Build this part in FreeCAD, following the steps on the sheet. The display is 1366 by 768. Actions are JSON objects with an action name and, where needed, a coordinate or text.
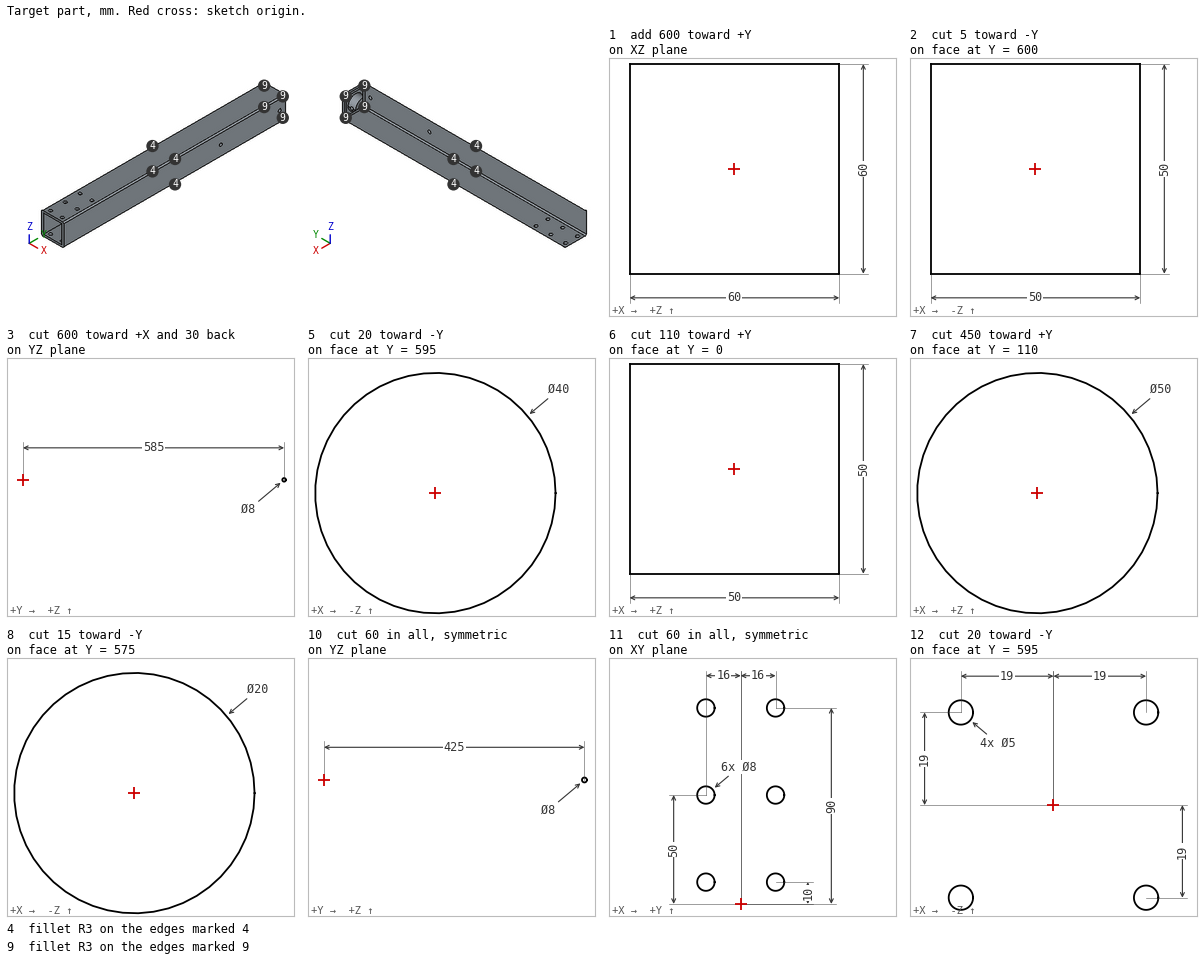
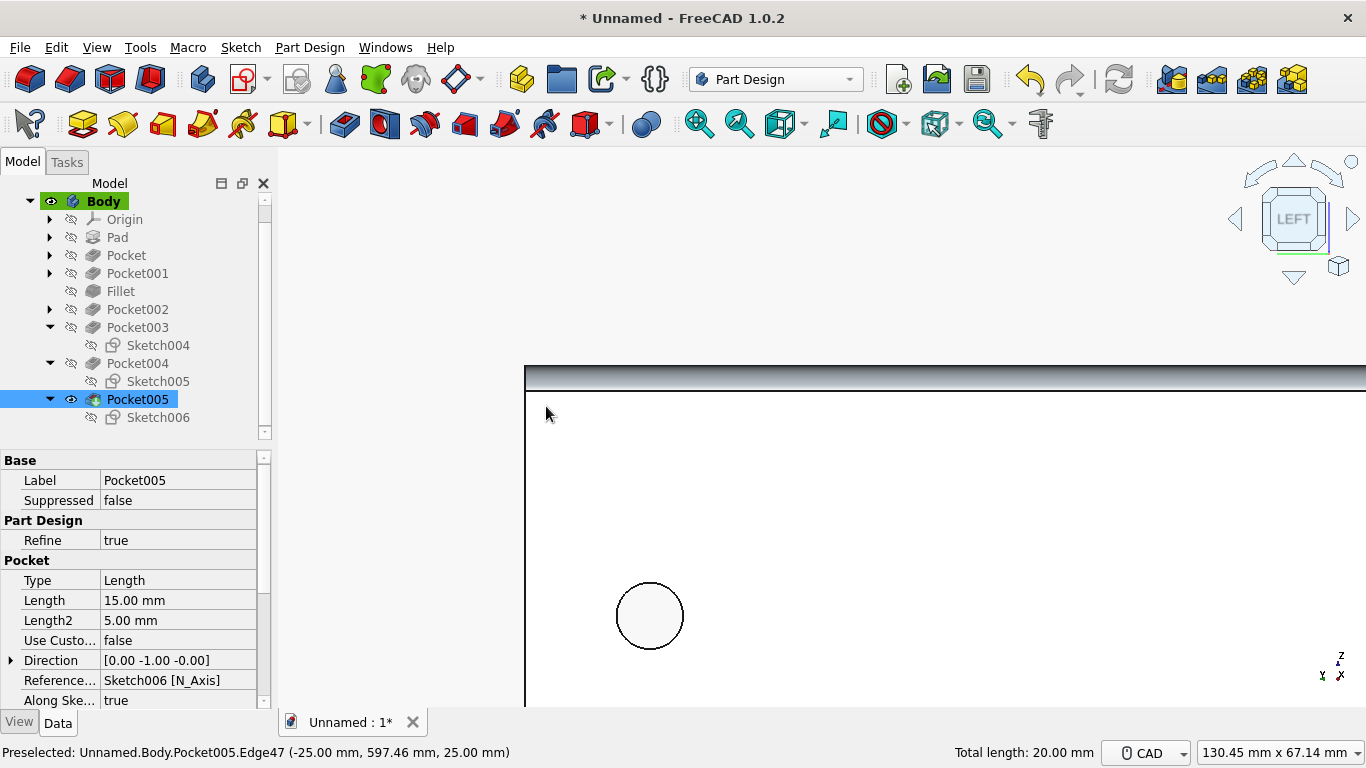
{"action": "left_click", "coordinate": [30, 80]}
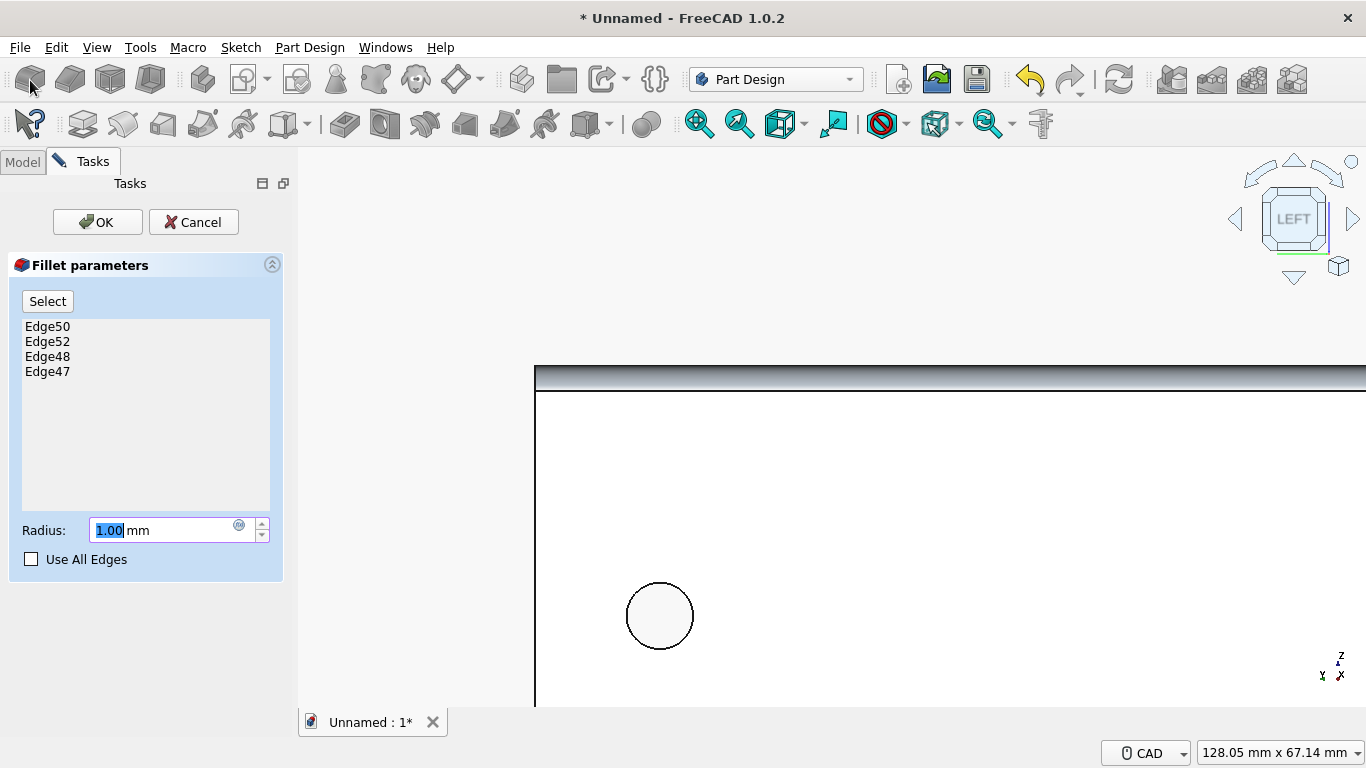
{"action": "type", "text": "3"}
{"action": "key", "text": "Tab"}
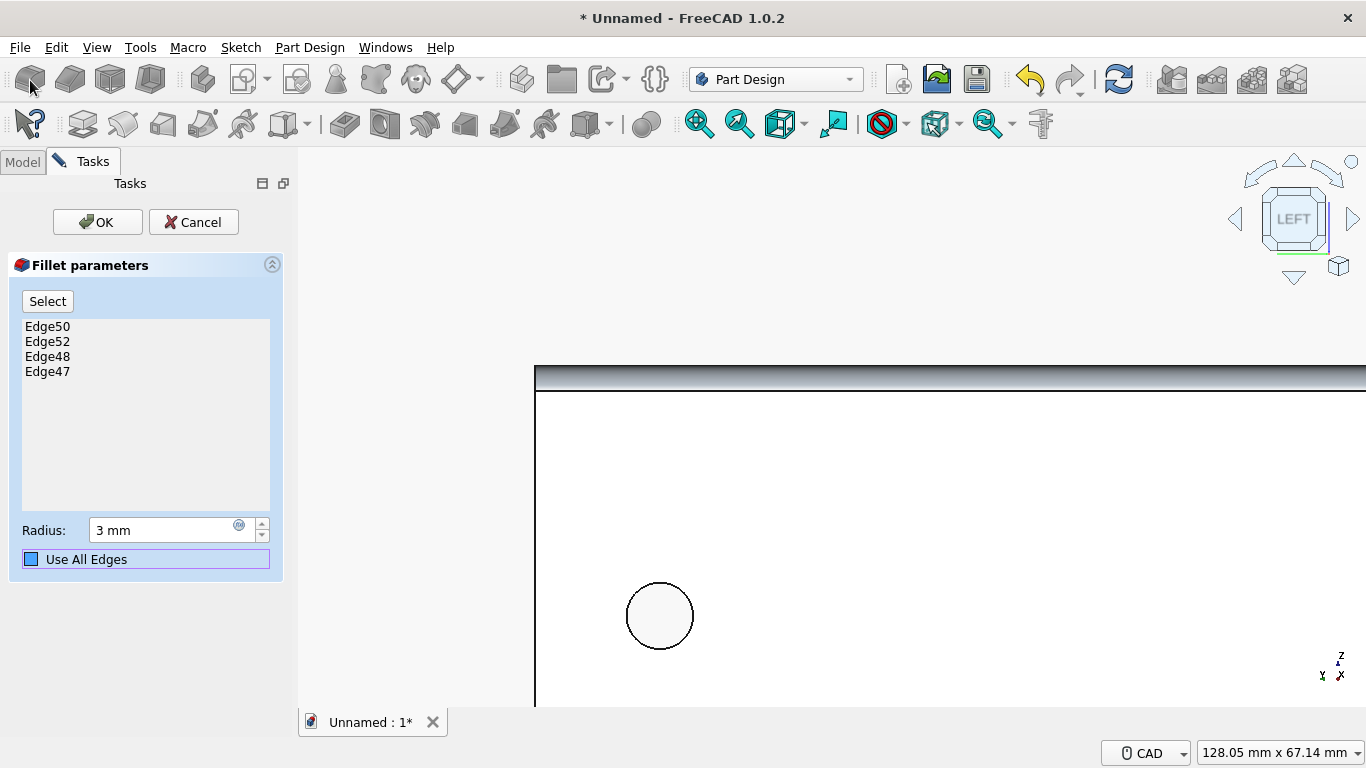
{"action": "left_click", "coordinate": [98, 222]}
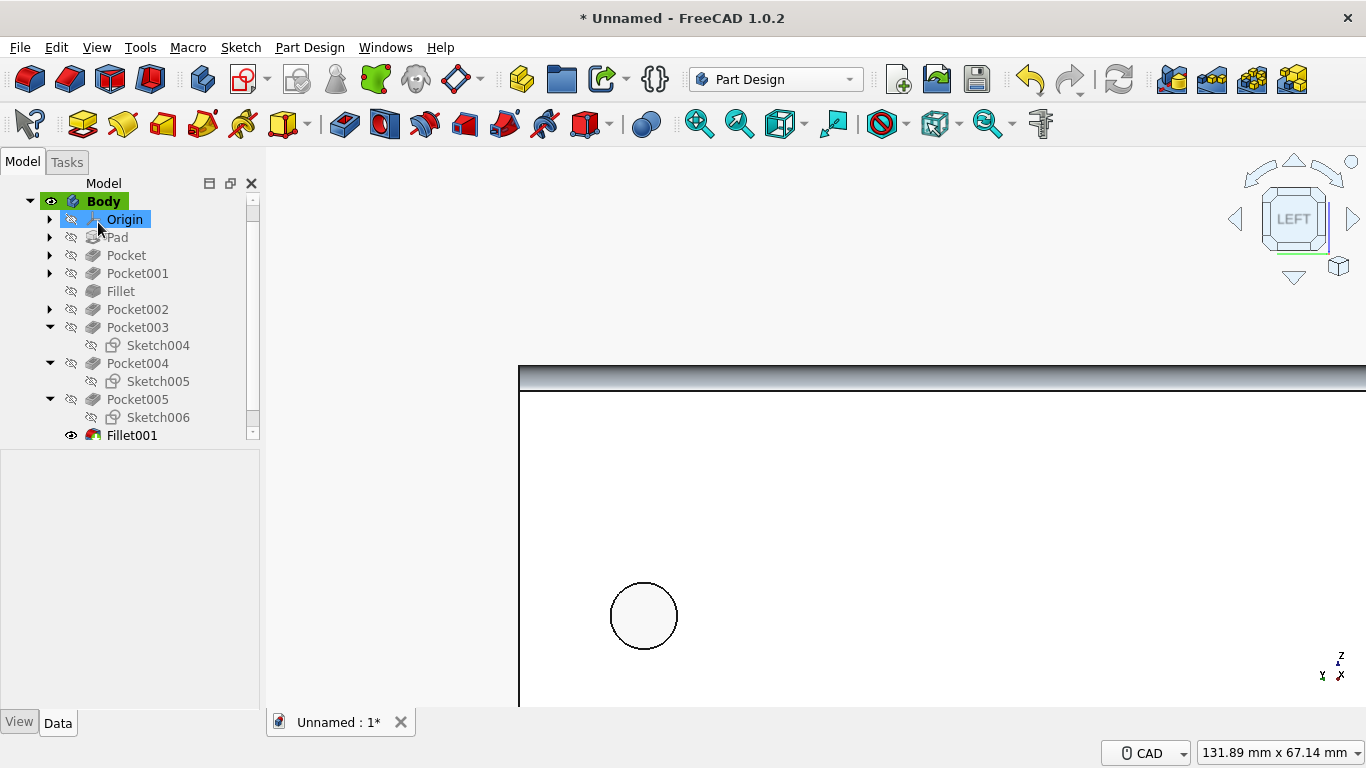
{"action": "key", "text": "v f"}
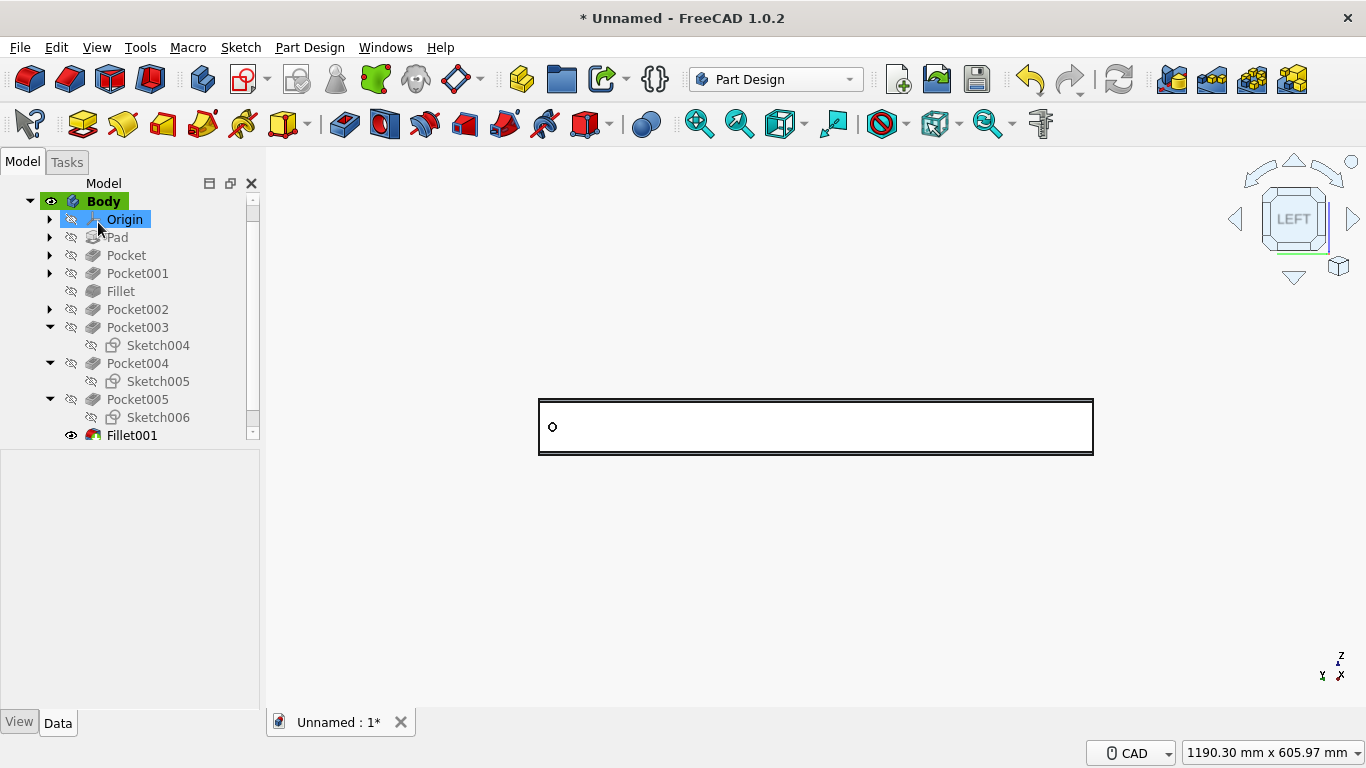
{"action": "left_click", "coordinate": [244, 80]}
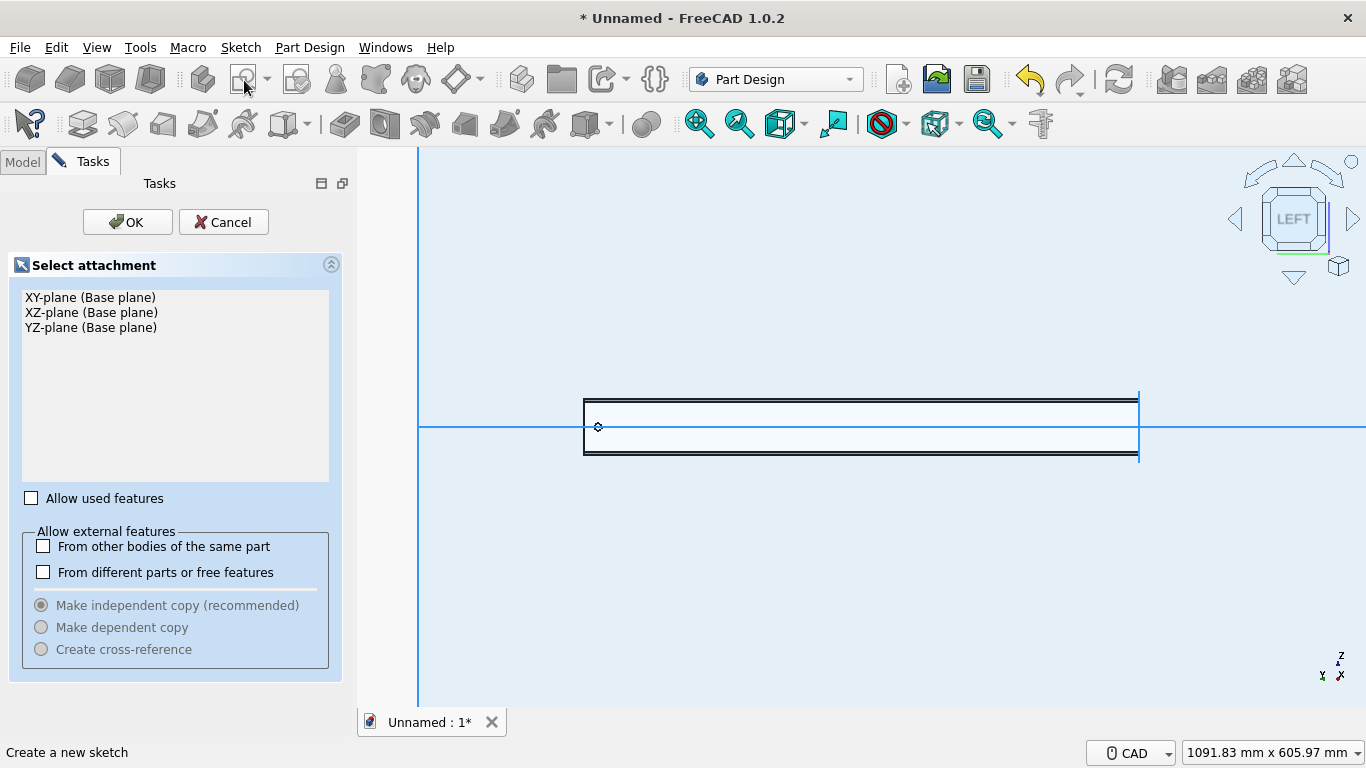
{"action": "left_click", "coordinate": [82, 328]}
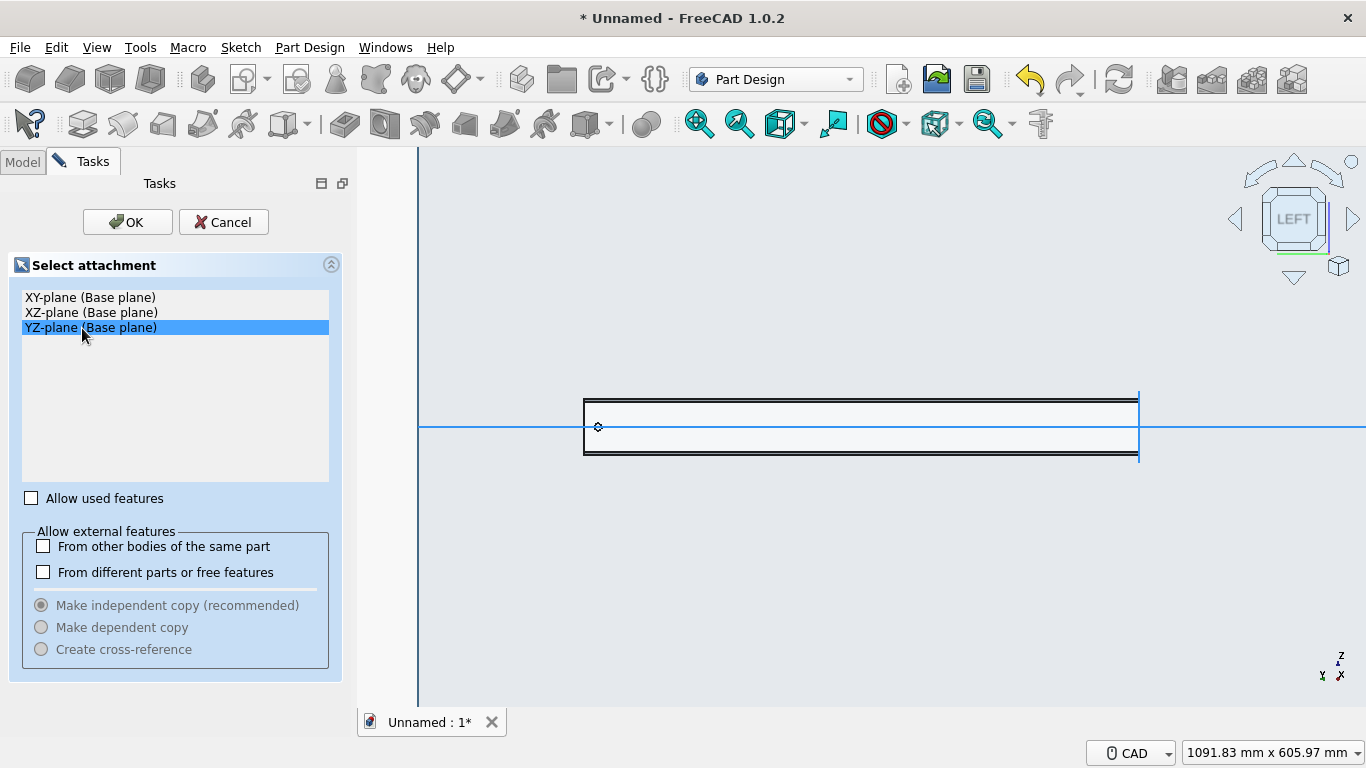
{"action": "left_click", "coordinate": [128, 222]}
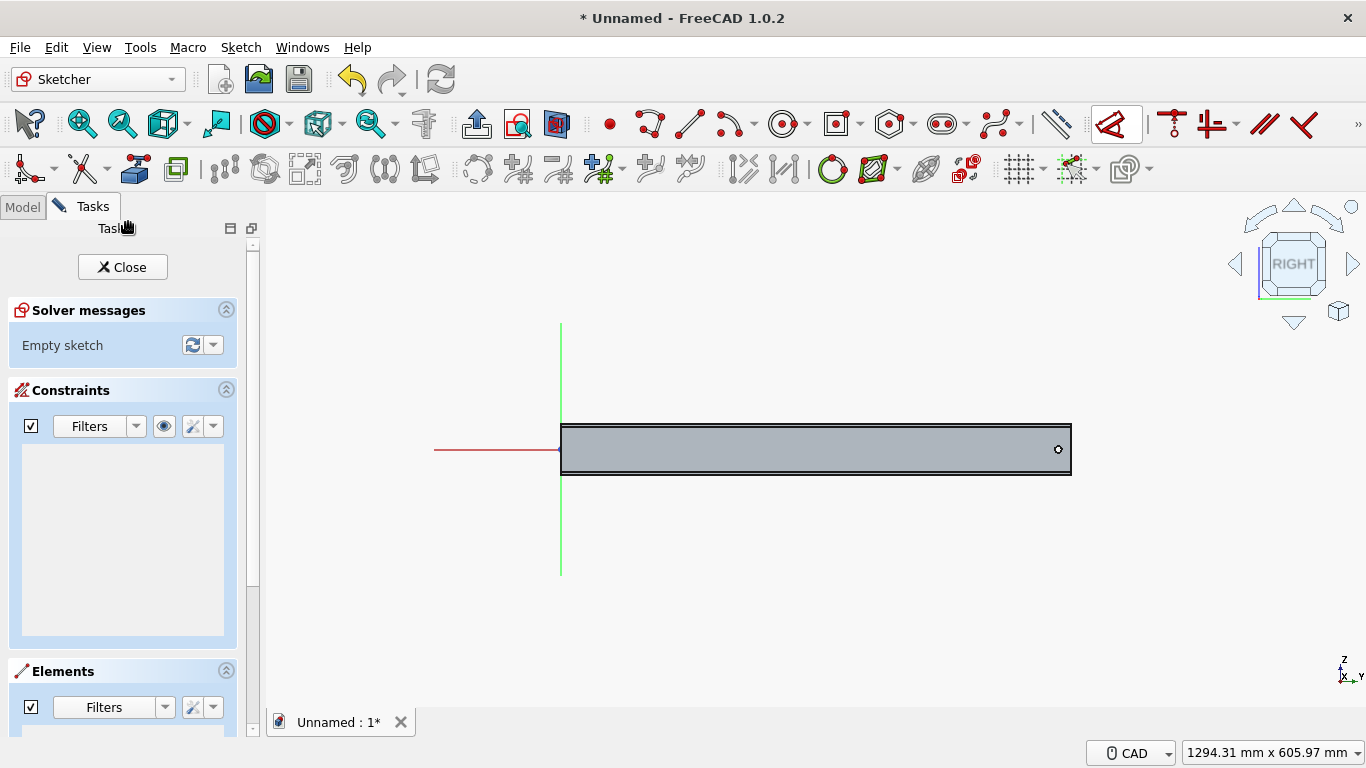
{"action": "key", "text": "q s"}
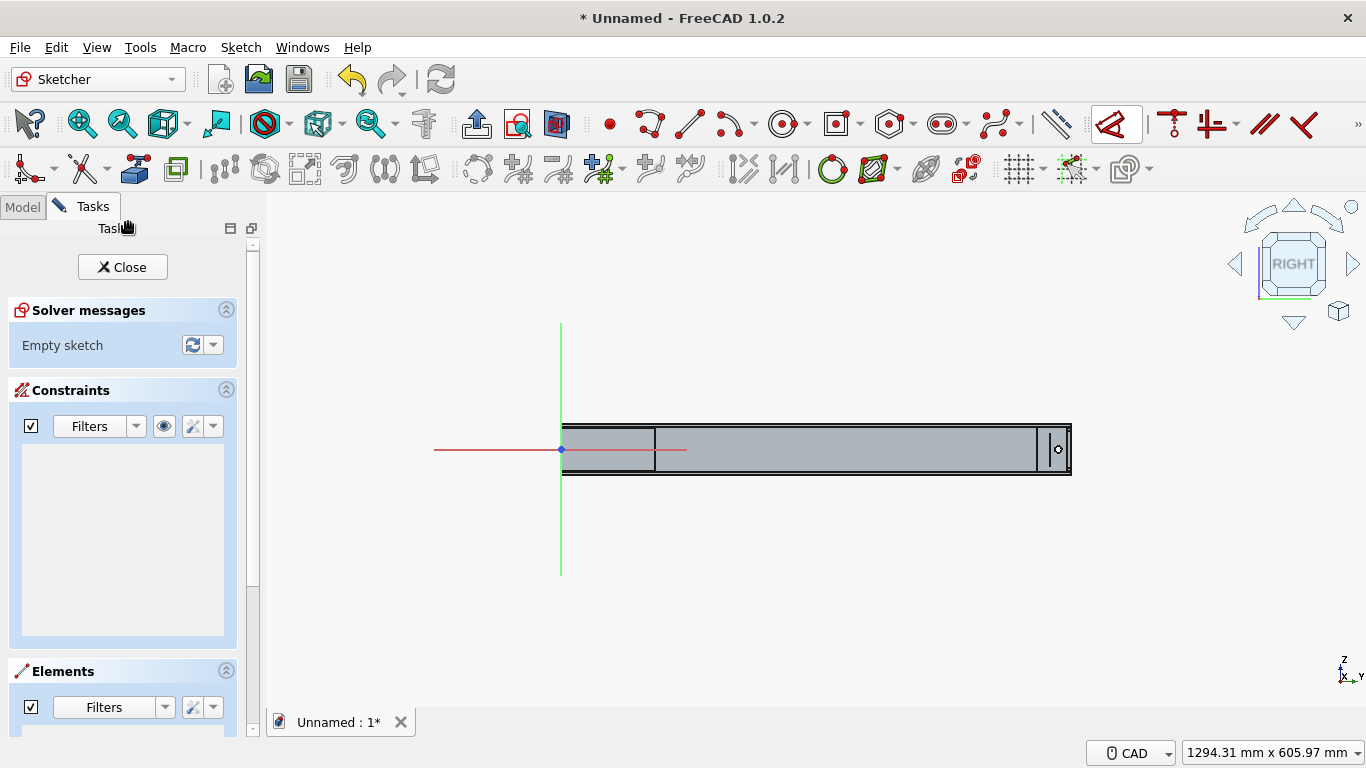
{"action": "scroll", "coordinate": [931, 450], "scroll_direction": "up", "scroll_amount": 15}